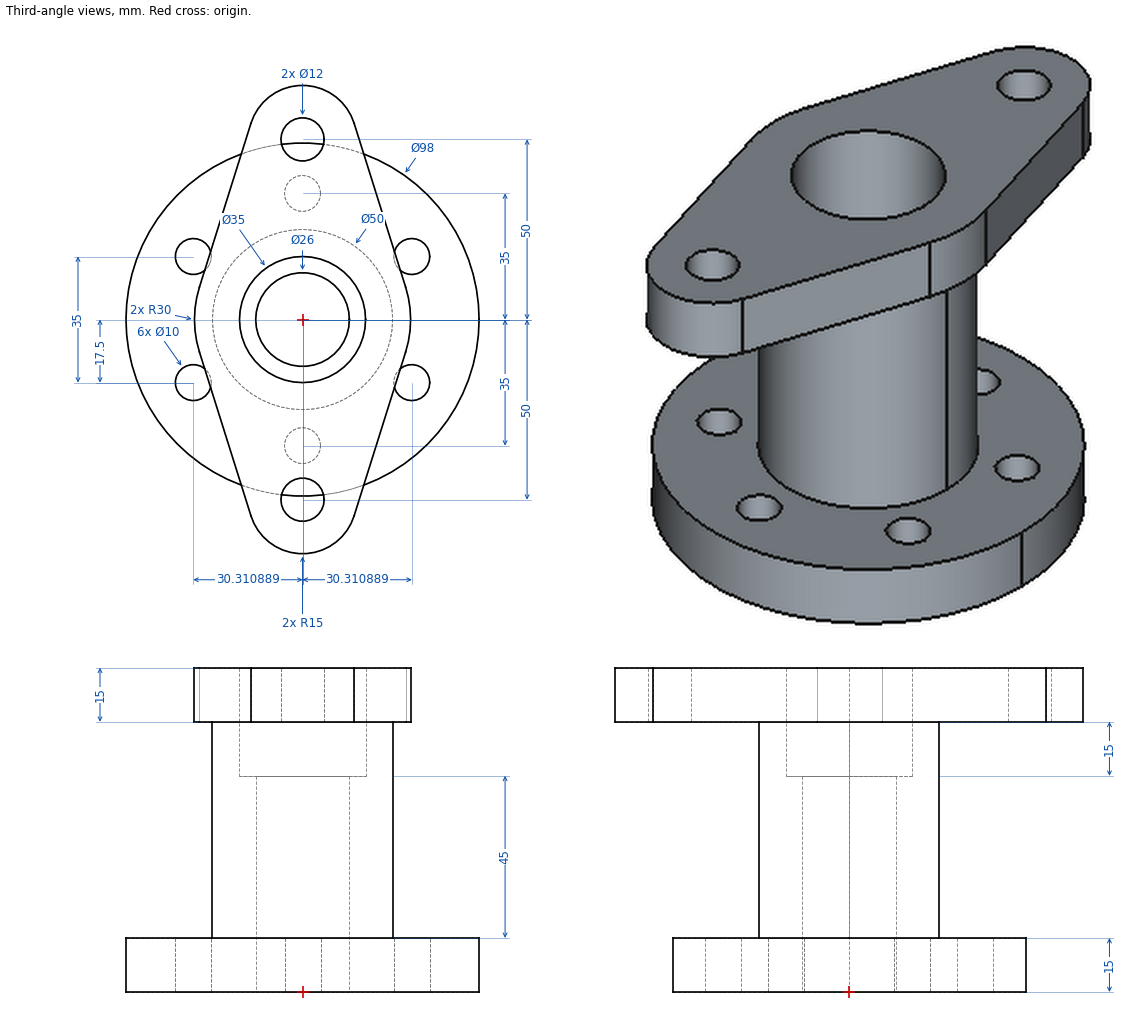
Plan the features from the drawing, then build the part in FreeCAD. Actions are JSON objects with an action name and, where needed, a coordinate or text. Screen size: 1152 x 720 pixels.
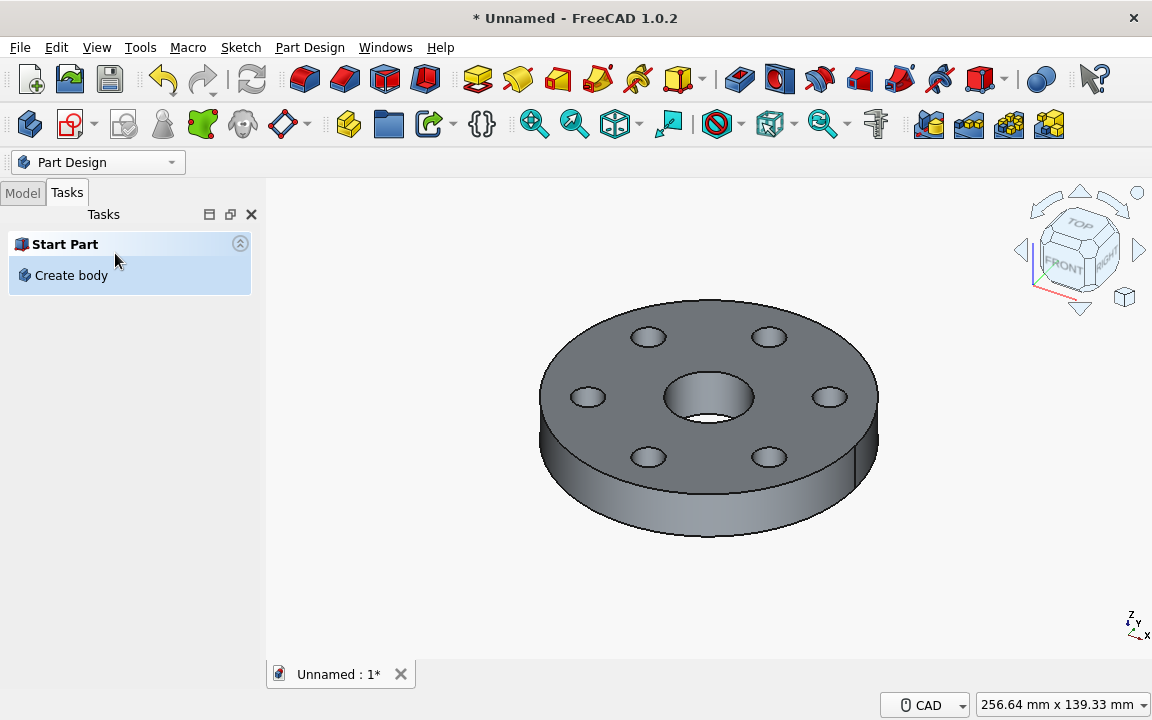
{"action": "left_click", "coordinate": [793, 424]}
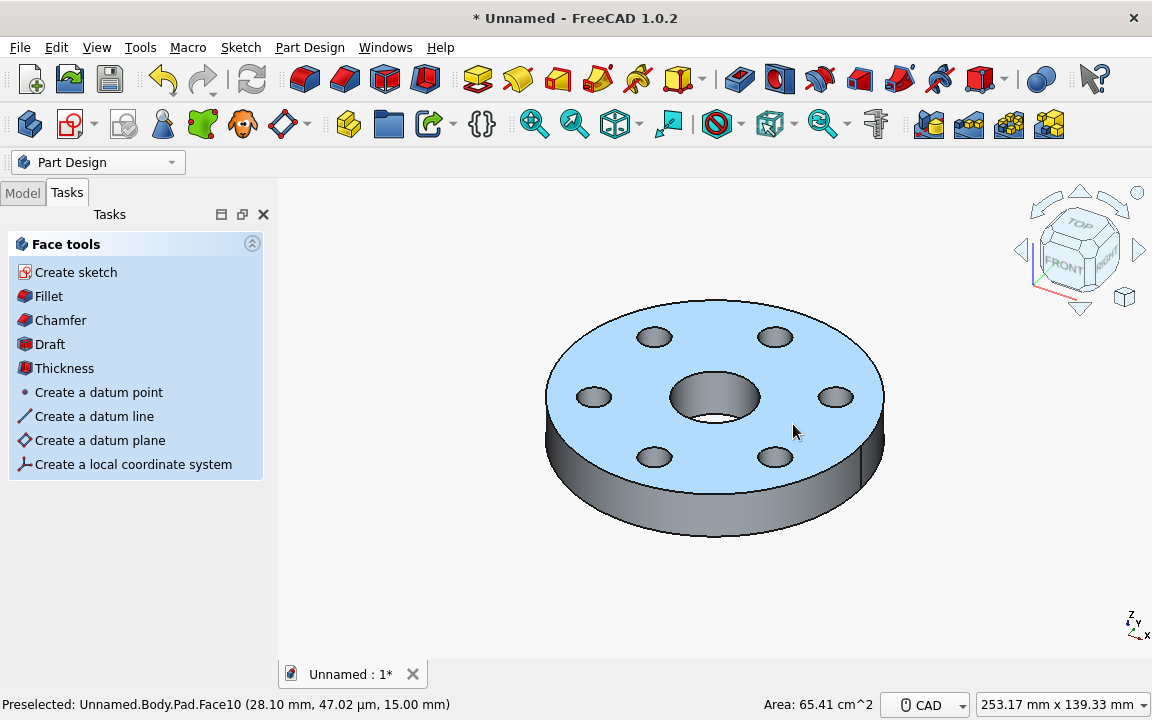
{"action": "left_click", "coordinate": [70, 124]}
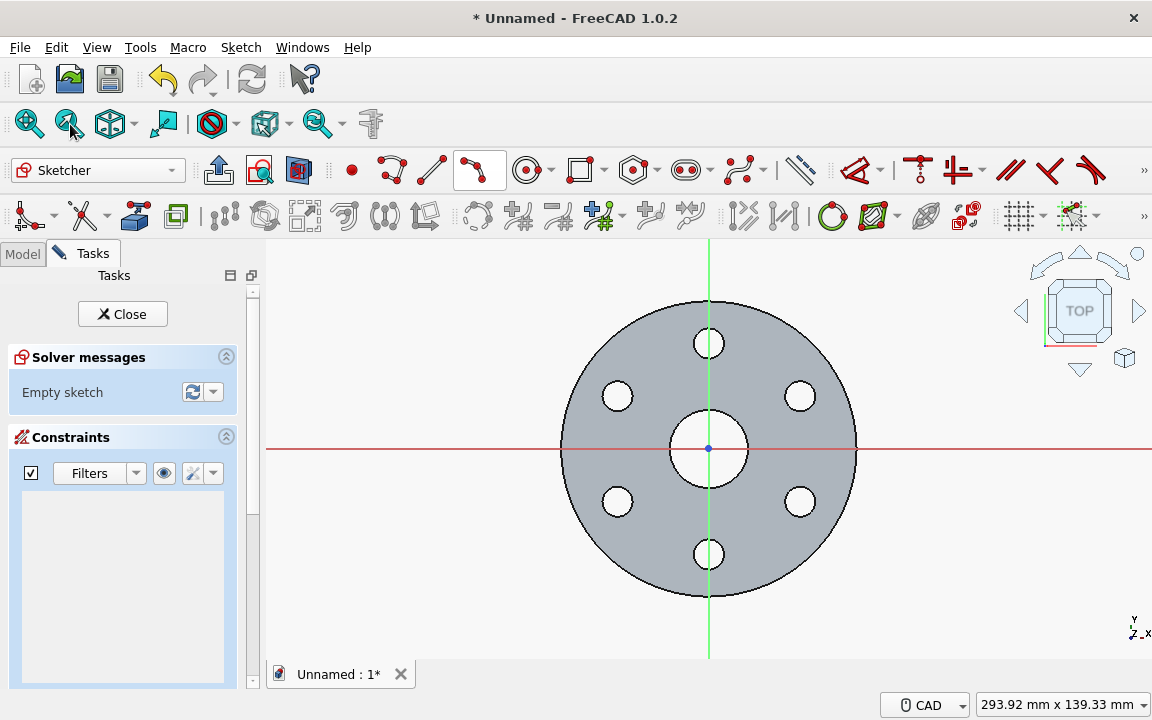
{"action": "scroll", "coordinate": [792, 449], "scroll_direction": "up", "scroll_amount": 3}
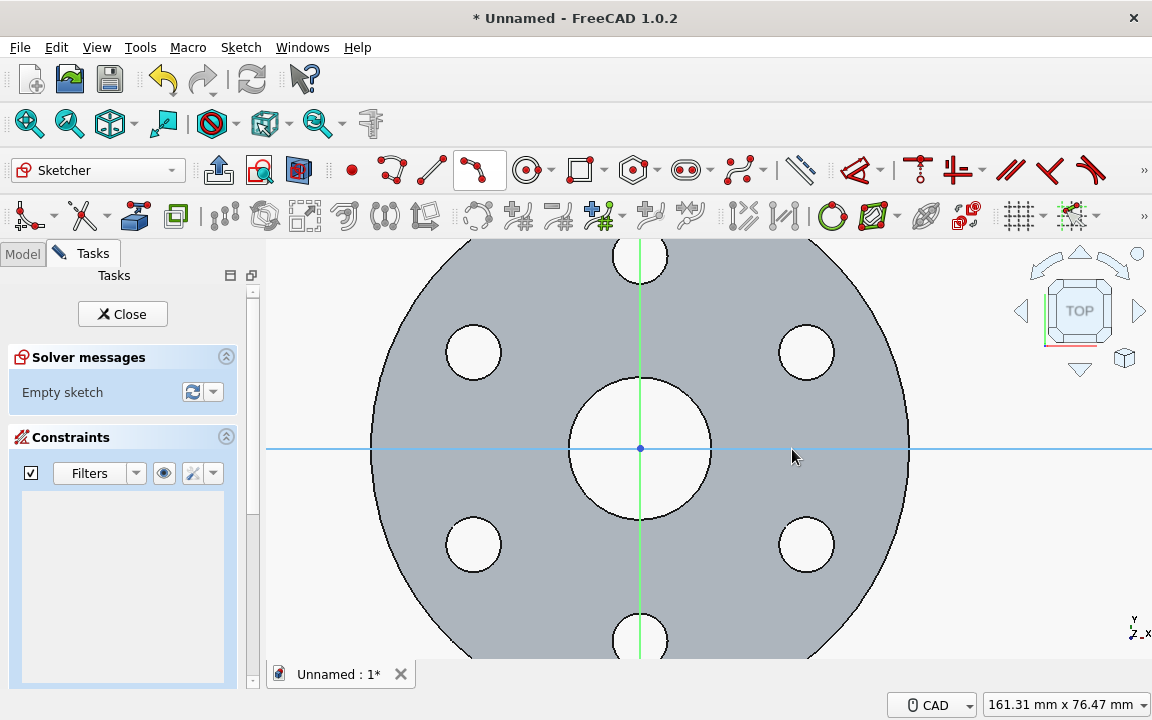
{"action": "left_click", "coordinate": [528, 170]}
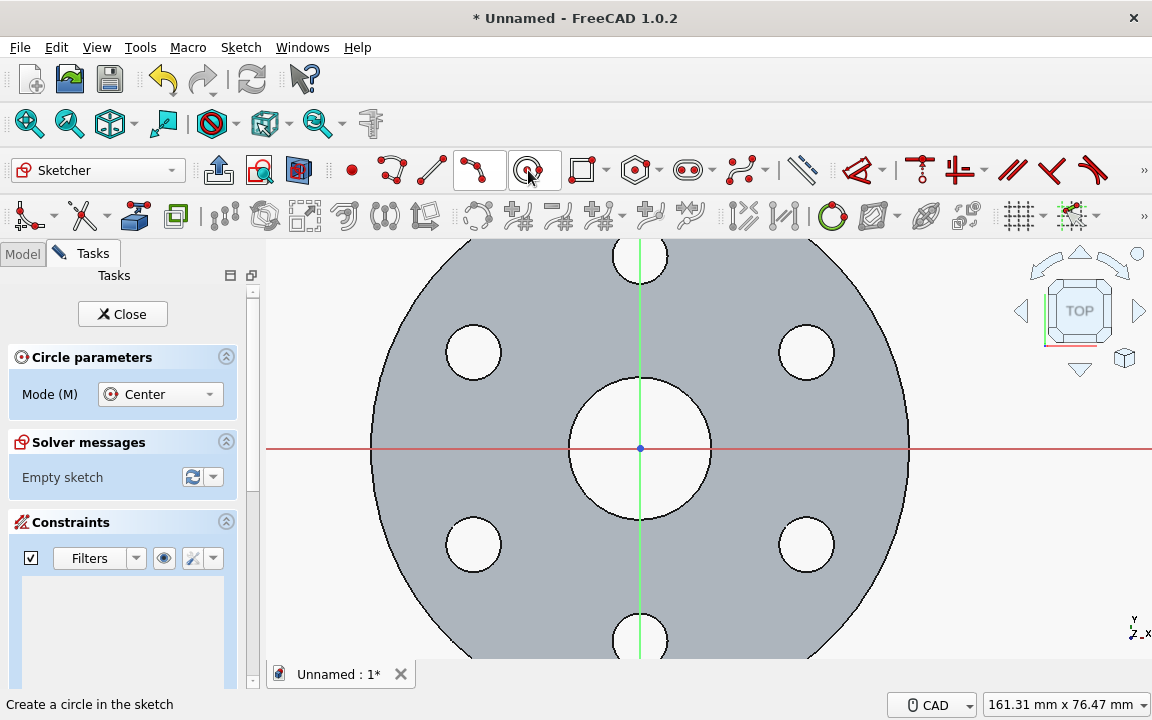
{"action": "left_click", "coordinate": [640, 449]}
{"action": "left_click", "coordinate": [737, 351]}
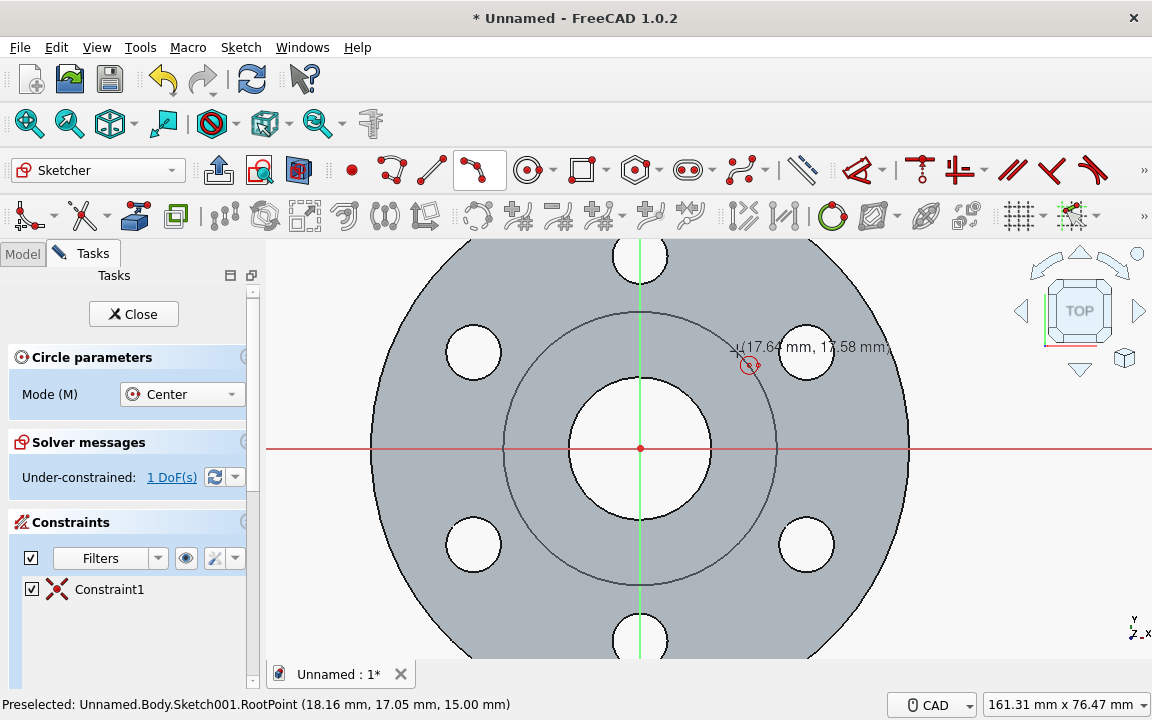
{"action": "left_click", "coordinate": [640, 449]}
{"action": "left_click", "coordinate": [691, 398]}
{"action": "key", "text": "Escape"}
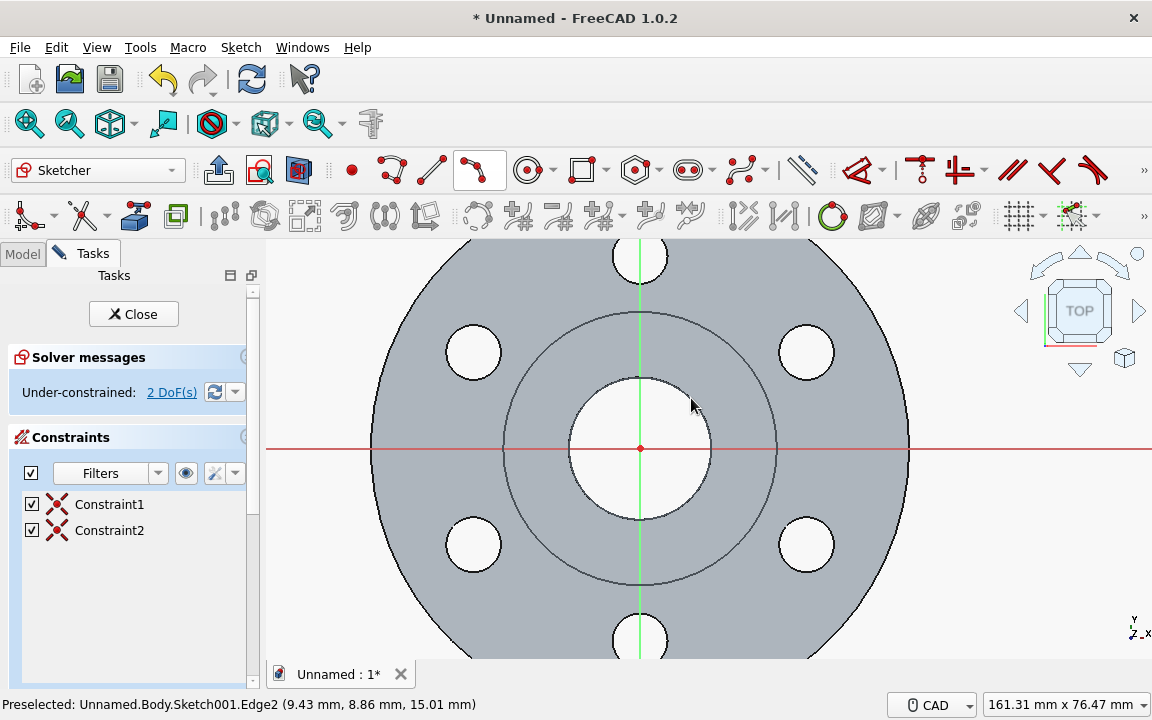
{"action": "left_click", "coordinate": [737, 352]}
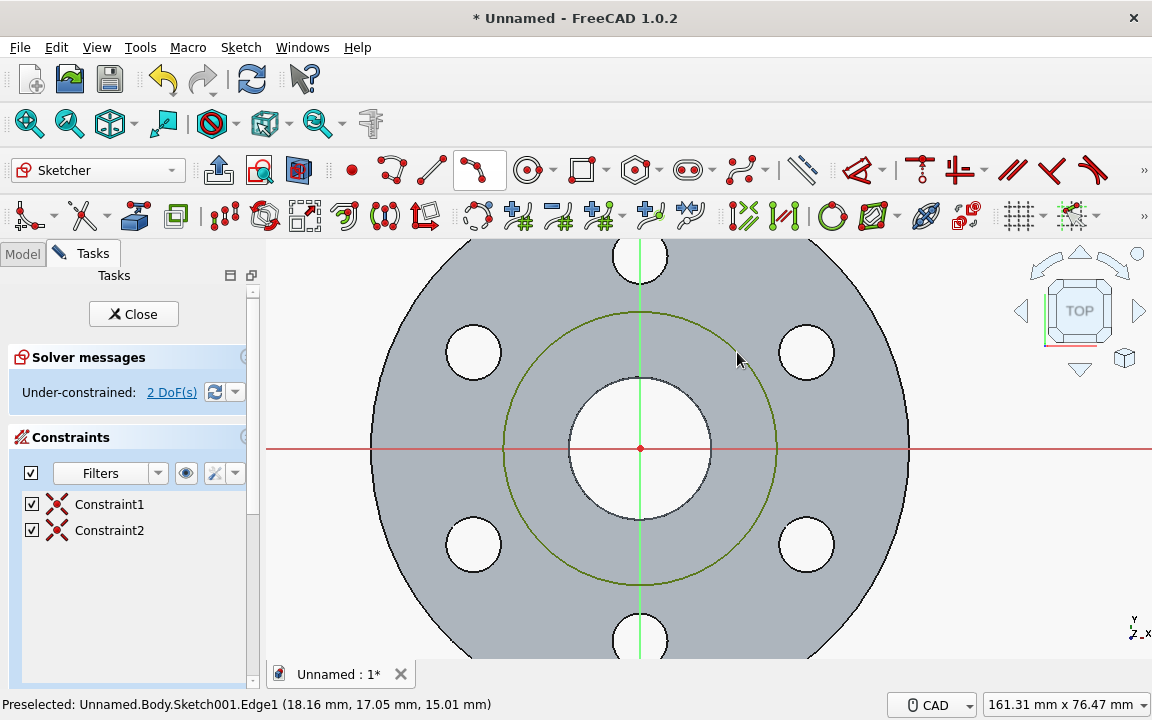
{"action": "left_click", "coordinate": [884, 170]}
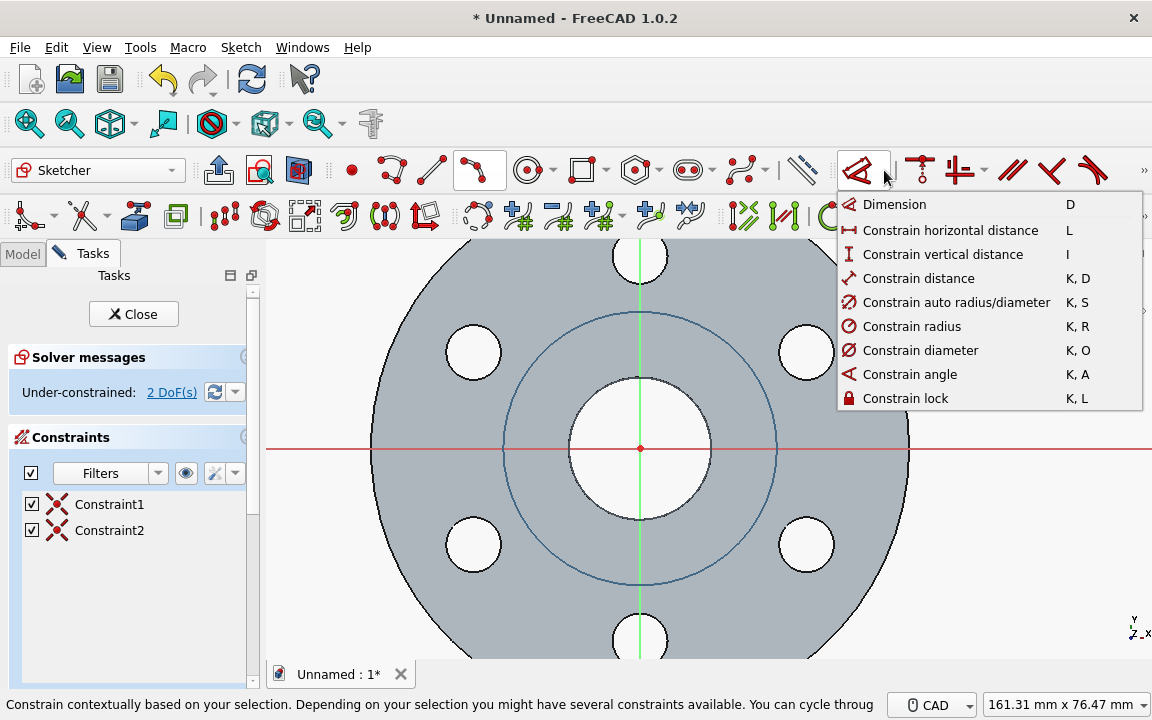
{"action": "left_click", "coordinate": [990, 350]}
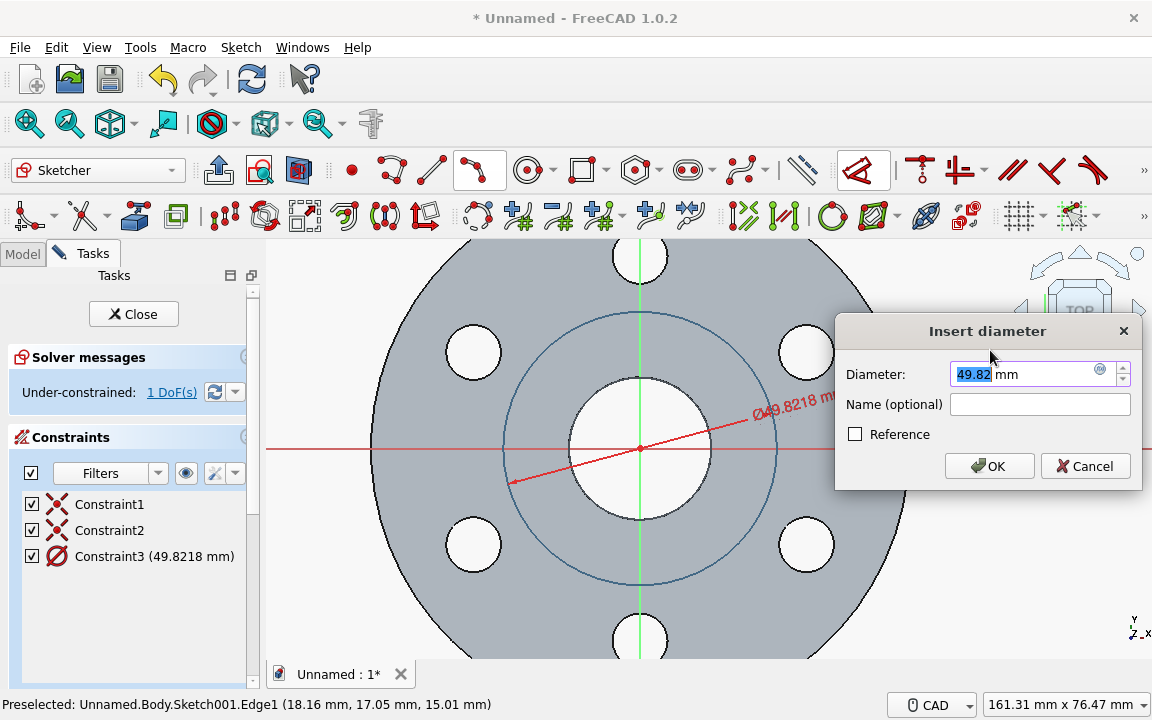
{"action": "type", "text": "50"}
{"action": "key", "text": "Return"}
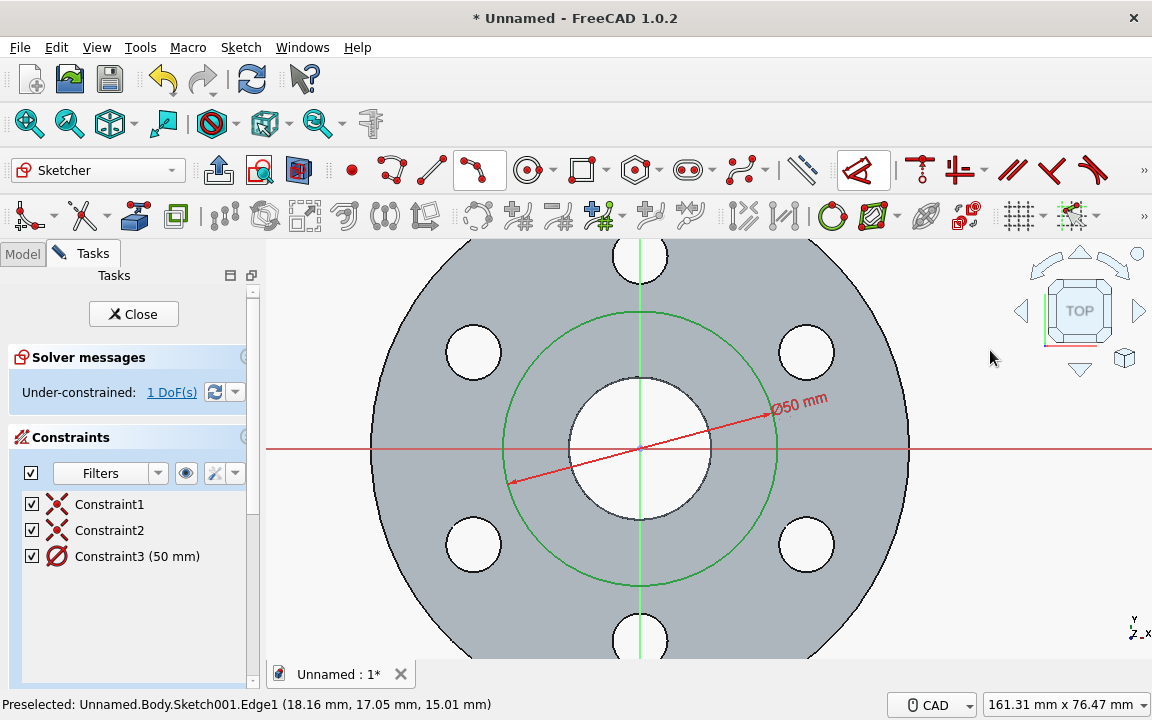
{"action": "left_click", "coordinate": [690, 398]}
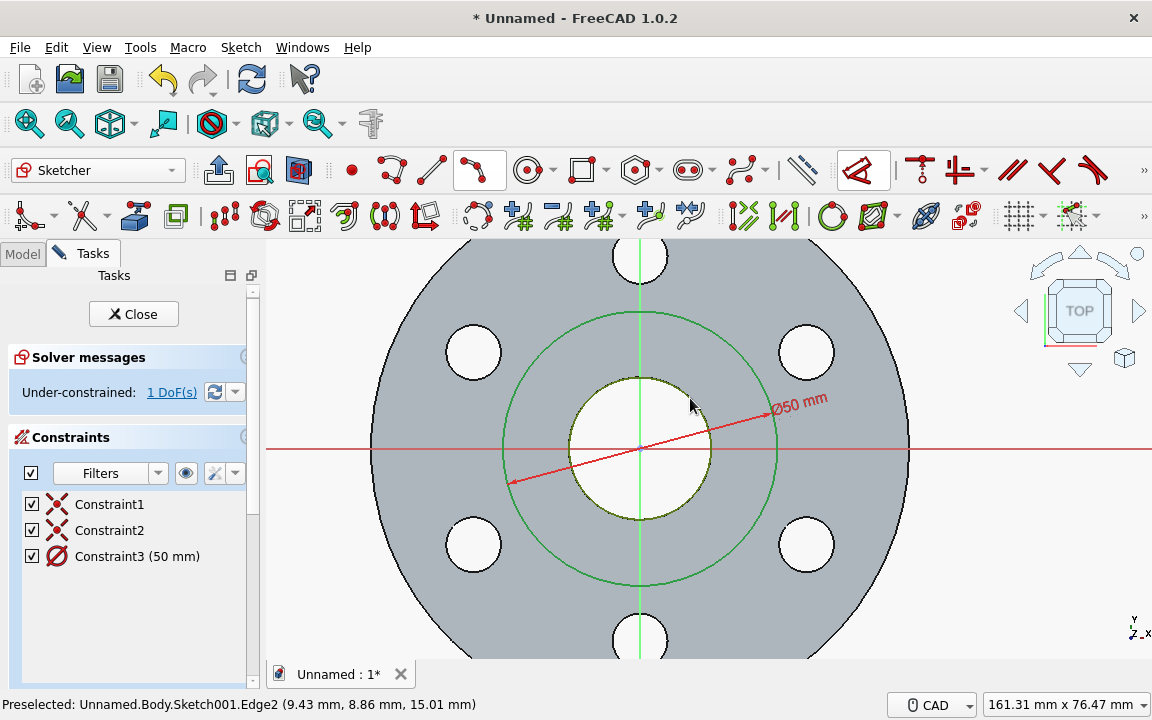
{"action": "key", "text": "k o"}